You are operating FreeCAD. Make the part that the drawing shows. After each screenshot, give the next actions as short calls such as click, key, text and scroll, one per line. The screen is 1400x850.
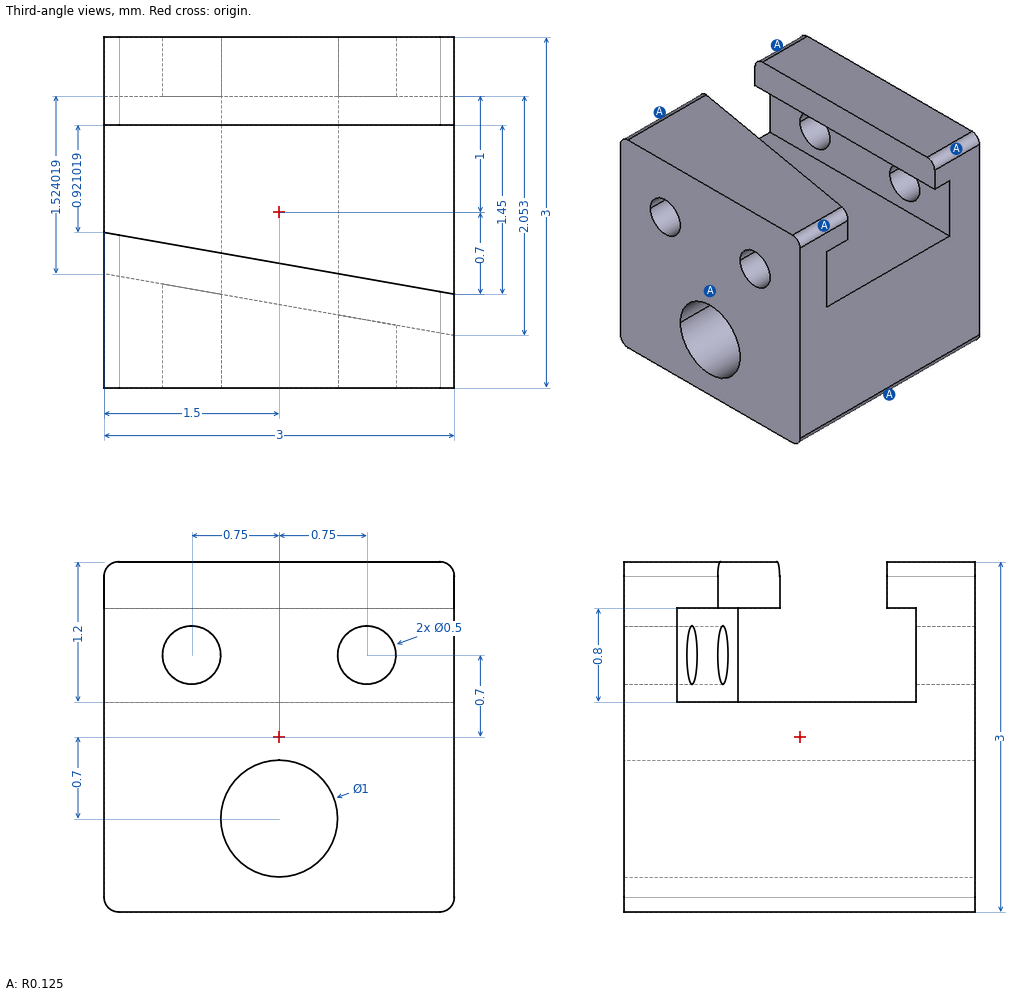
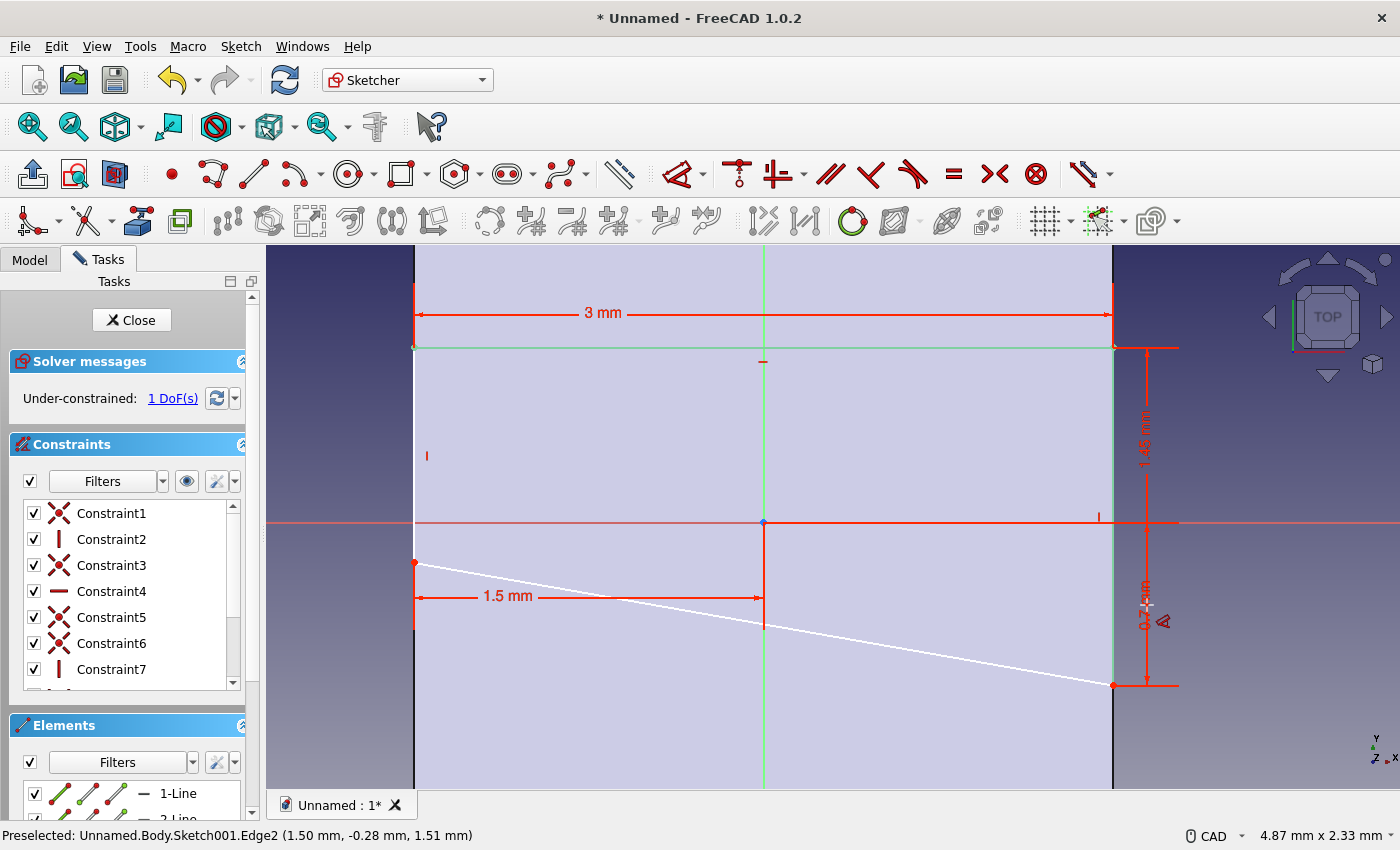
click(414, 412)
click(380, 455)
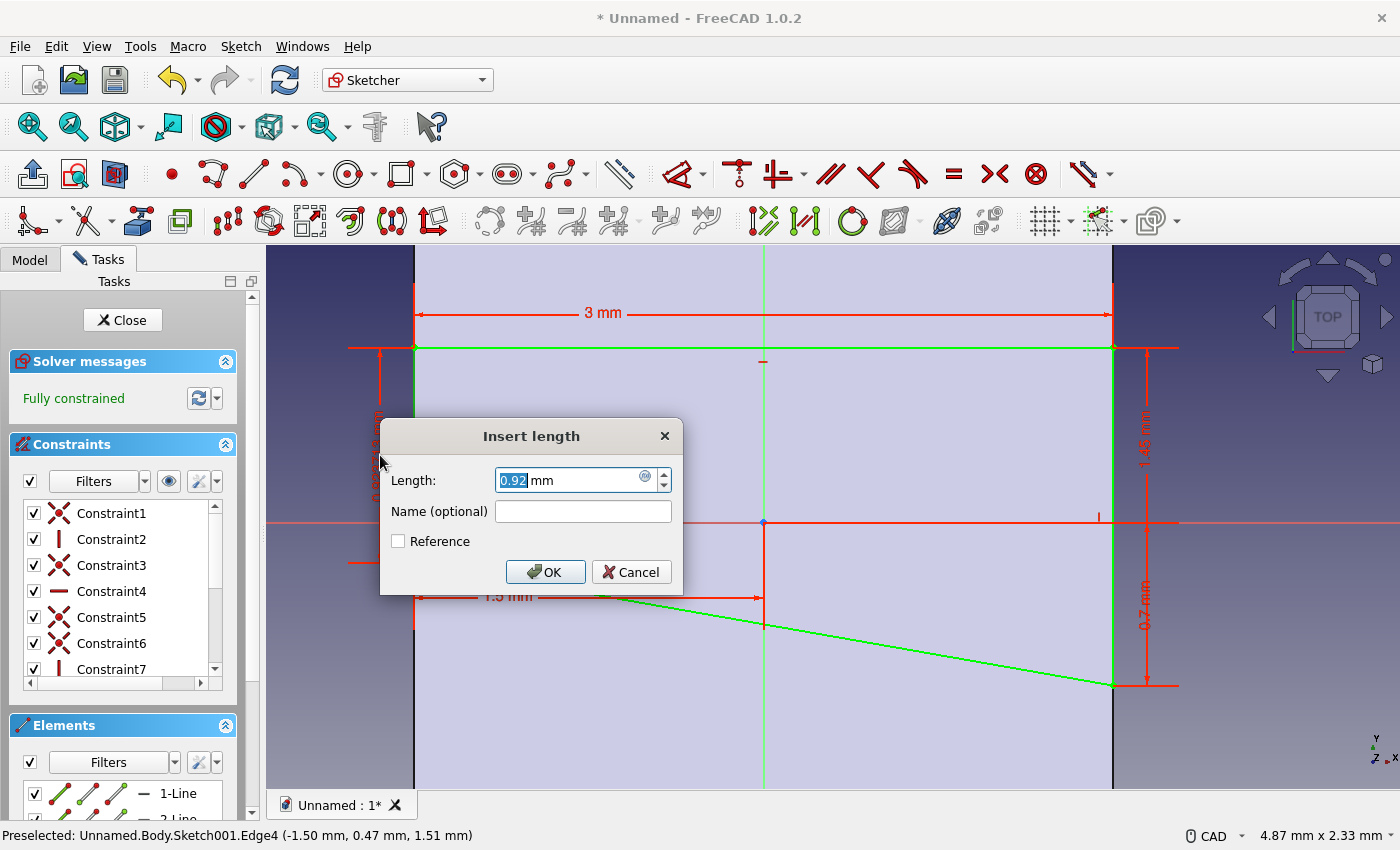
text(0.921019)
key(Return)
key(Escape)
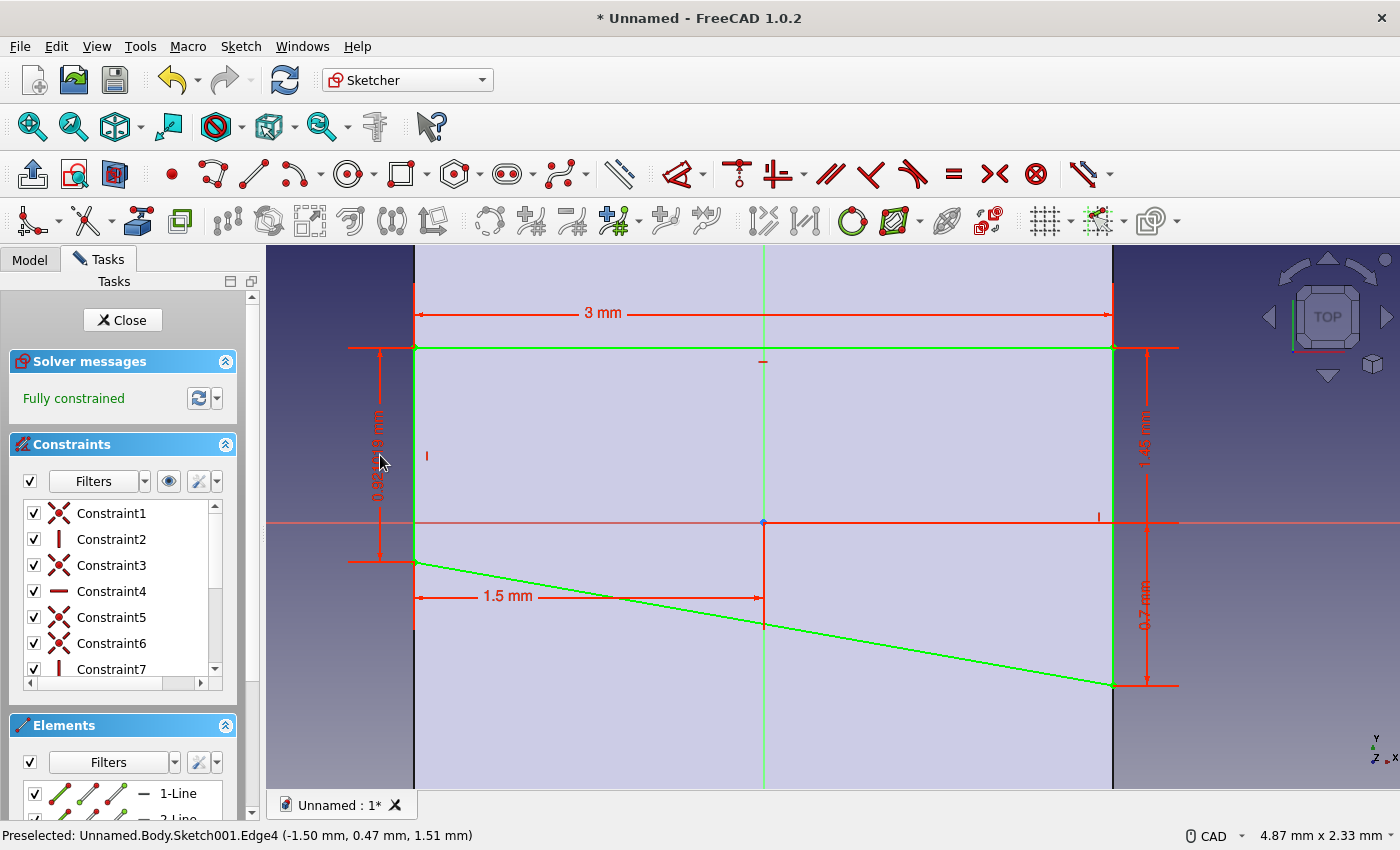
click(123, 320)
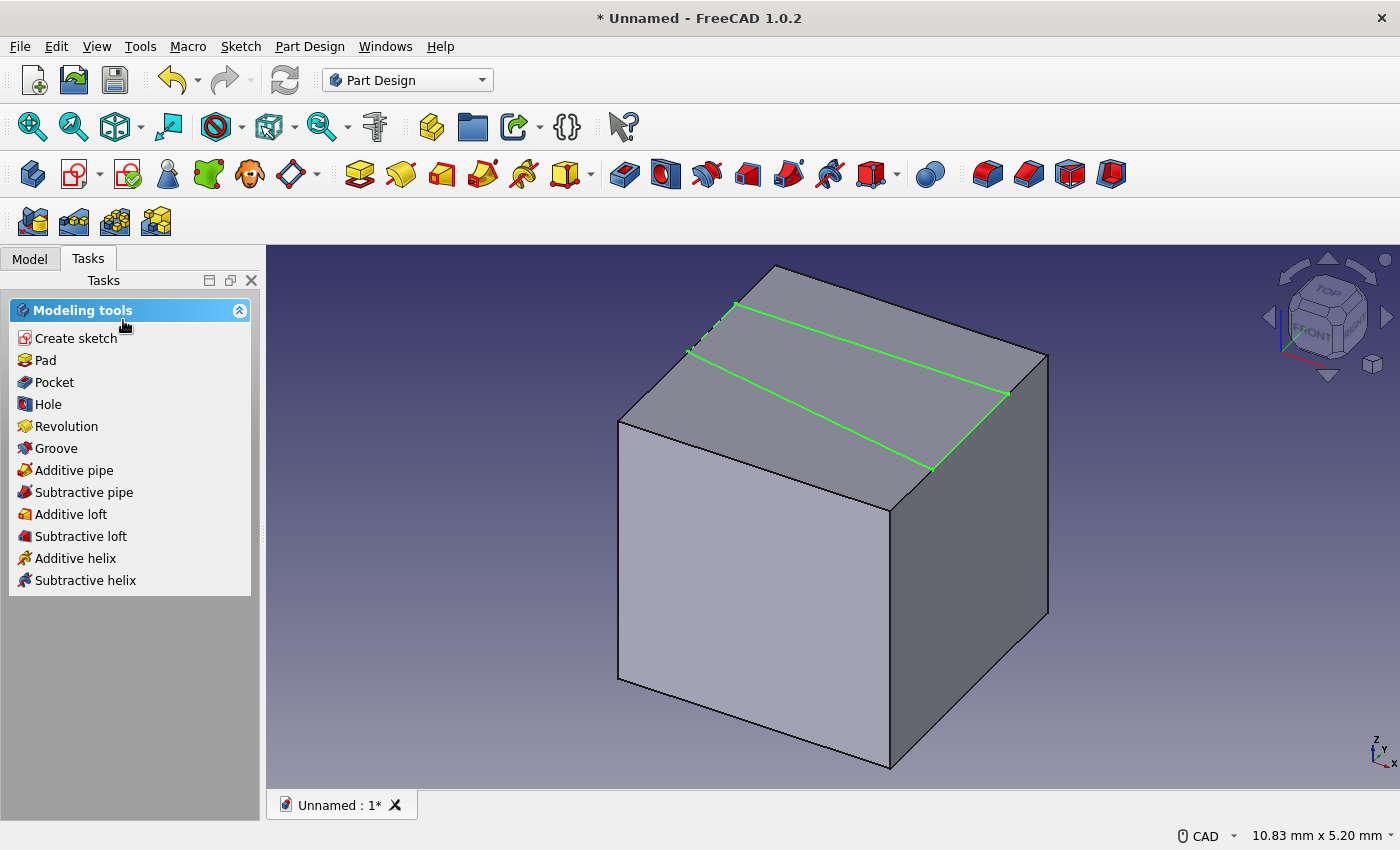
click(625, 174)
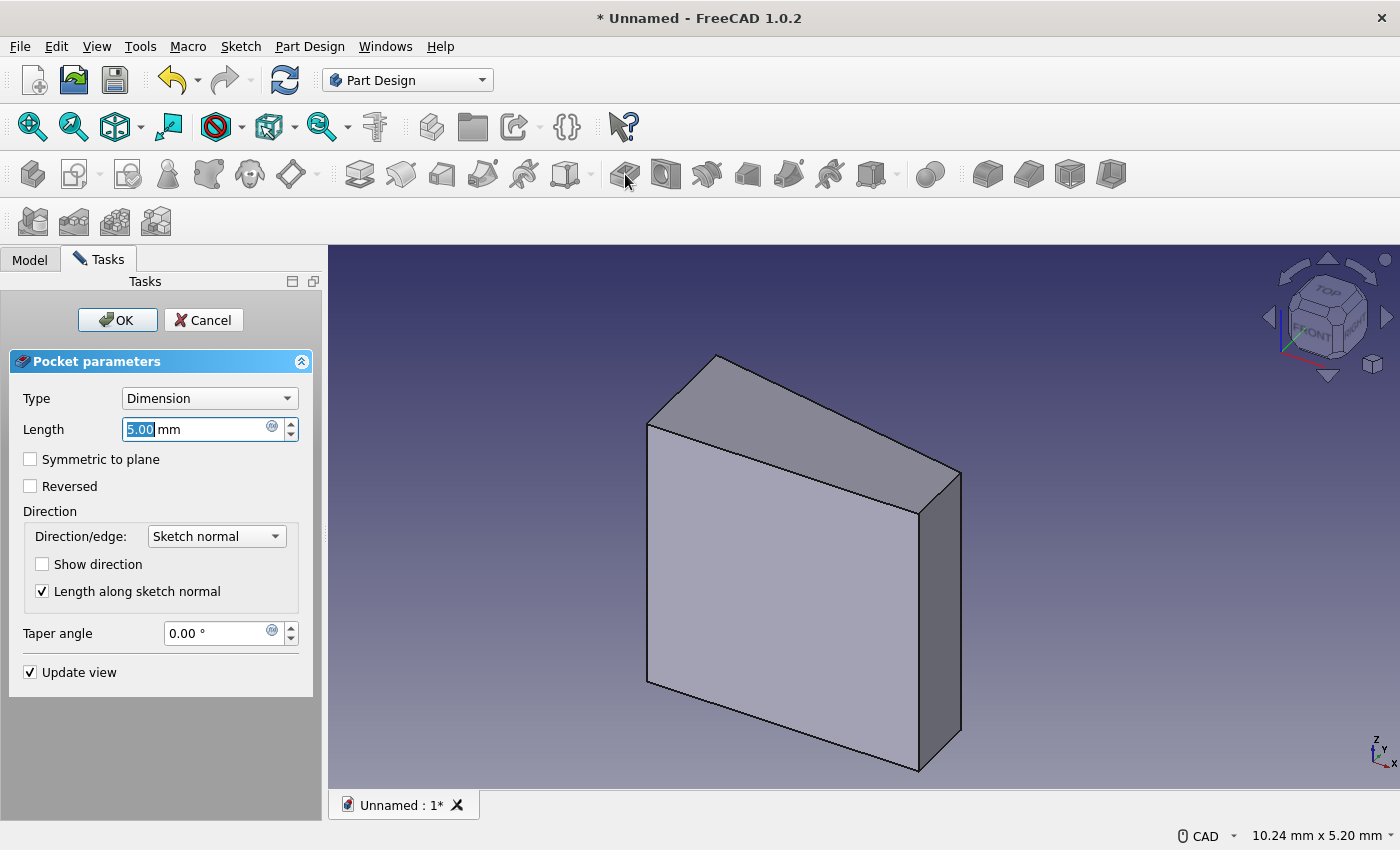
text(1.2)
key(Tab)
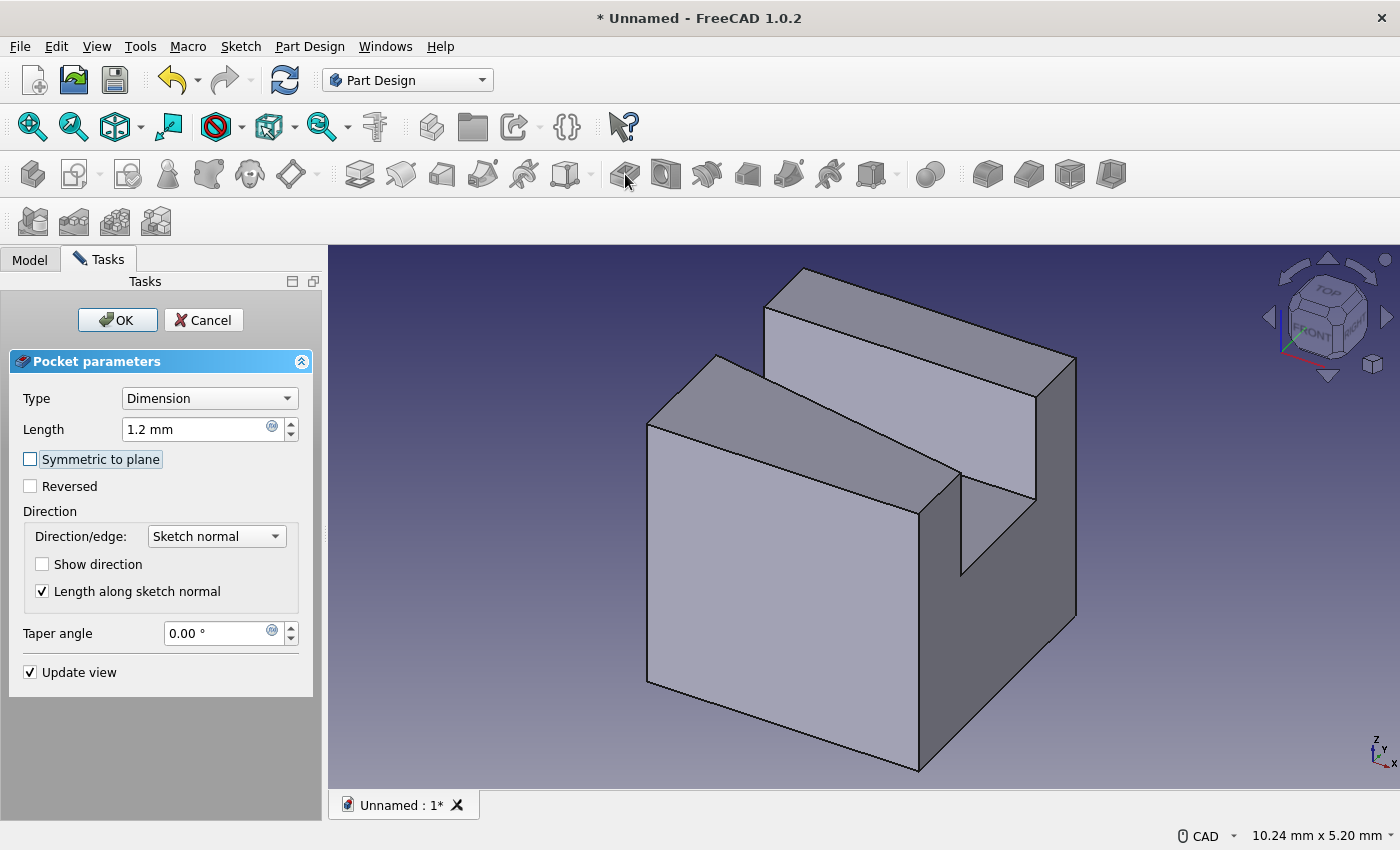
click(118, 320)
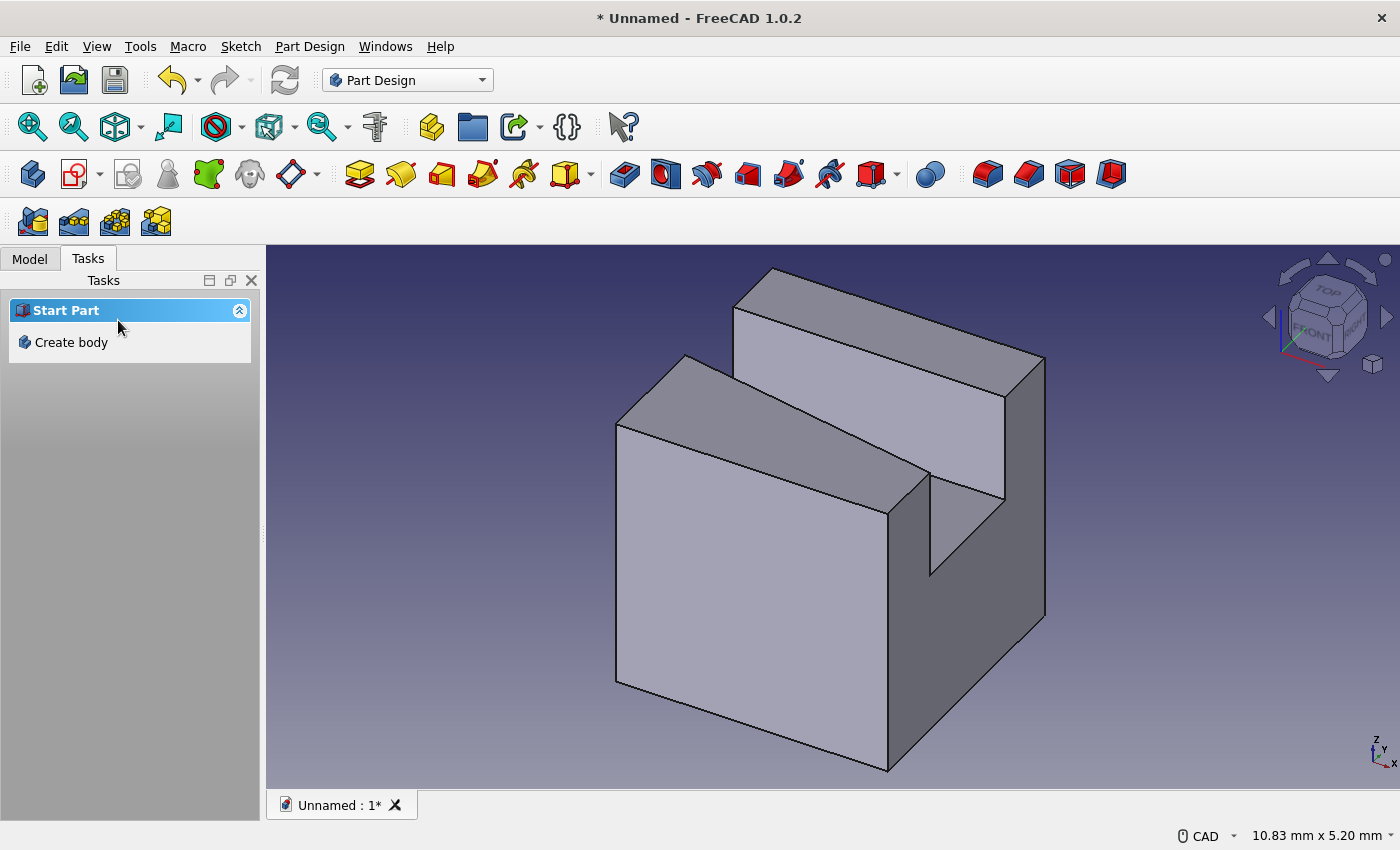
key(0)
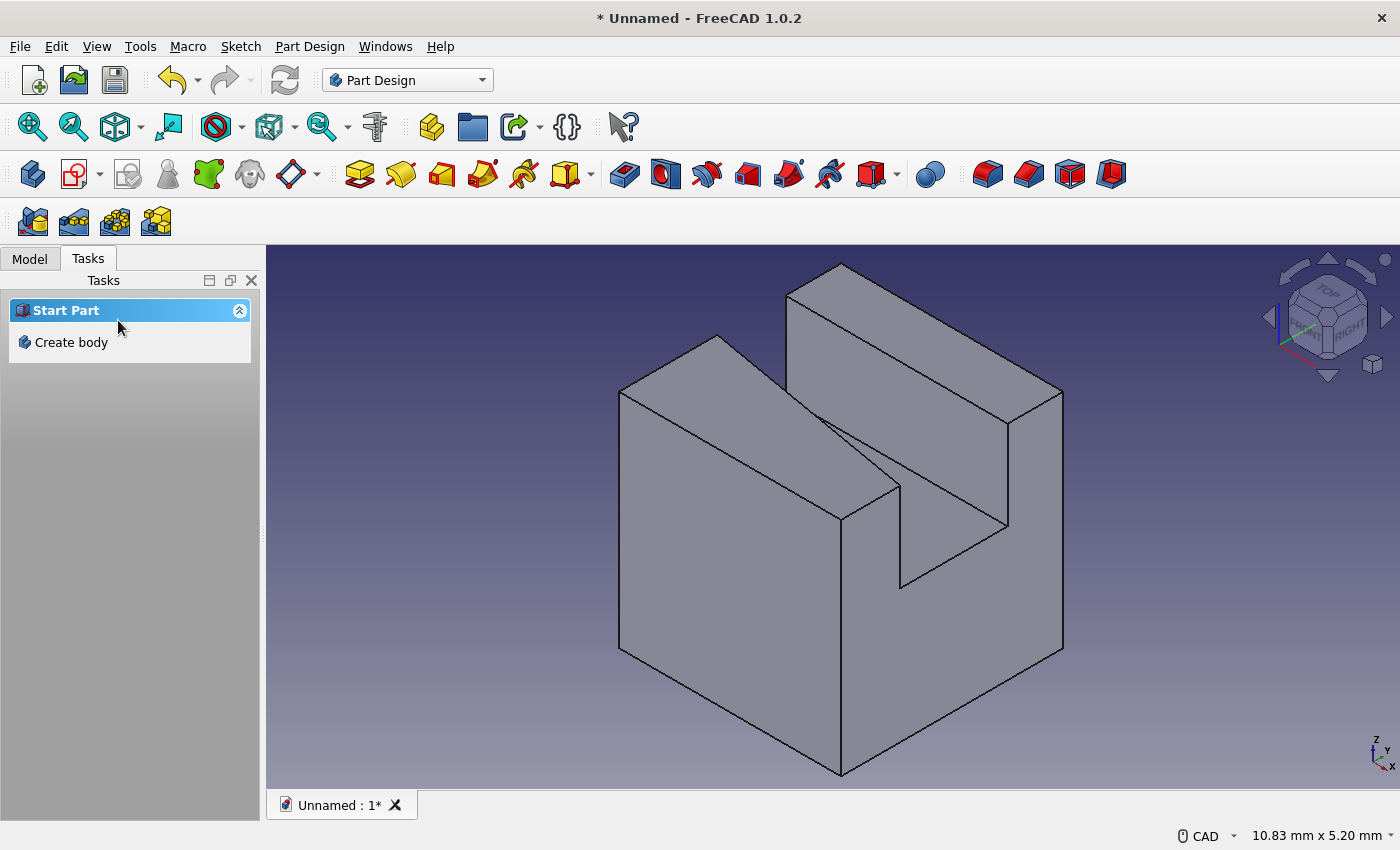
click(922, 520)